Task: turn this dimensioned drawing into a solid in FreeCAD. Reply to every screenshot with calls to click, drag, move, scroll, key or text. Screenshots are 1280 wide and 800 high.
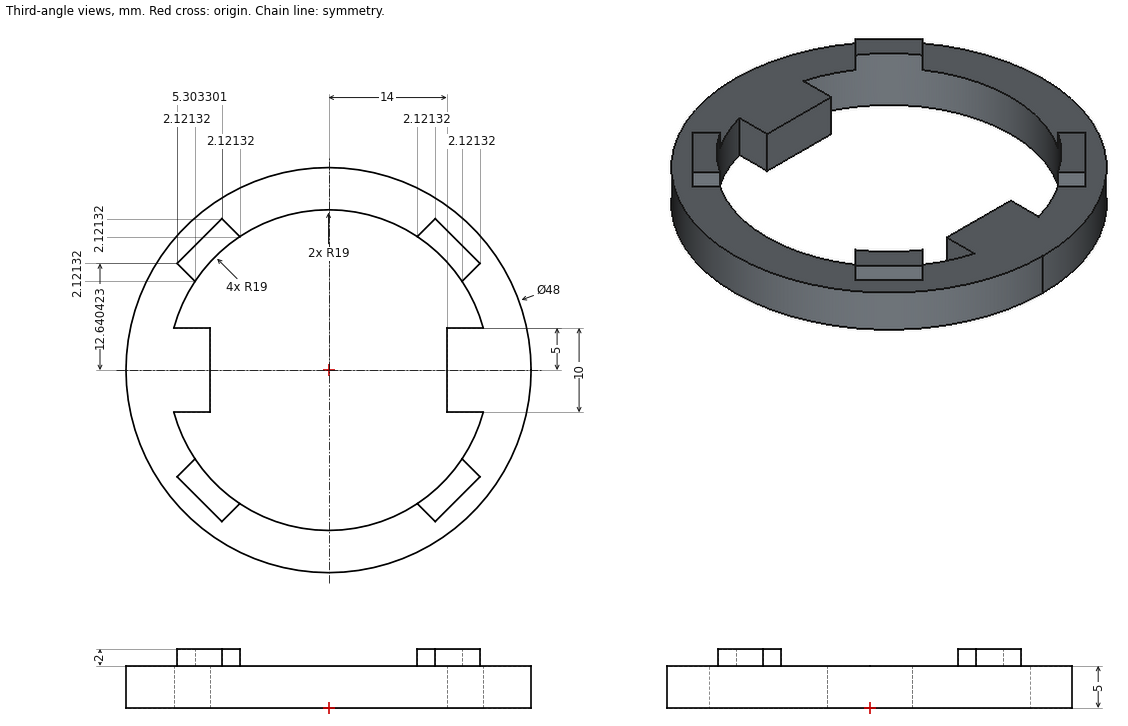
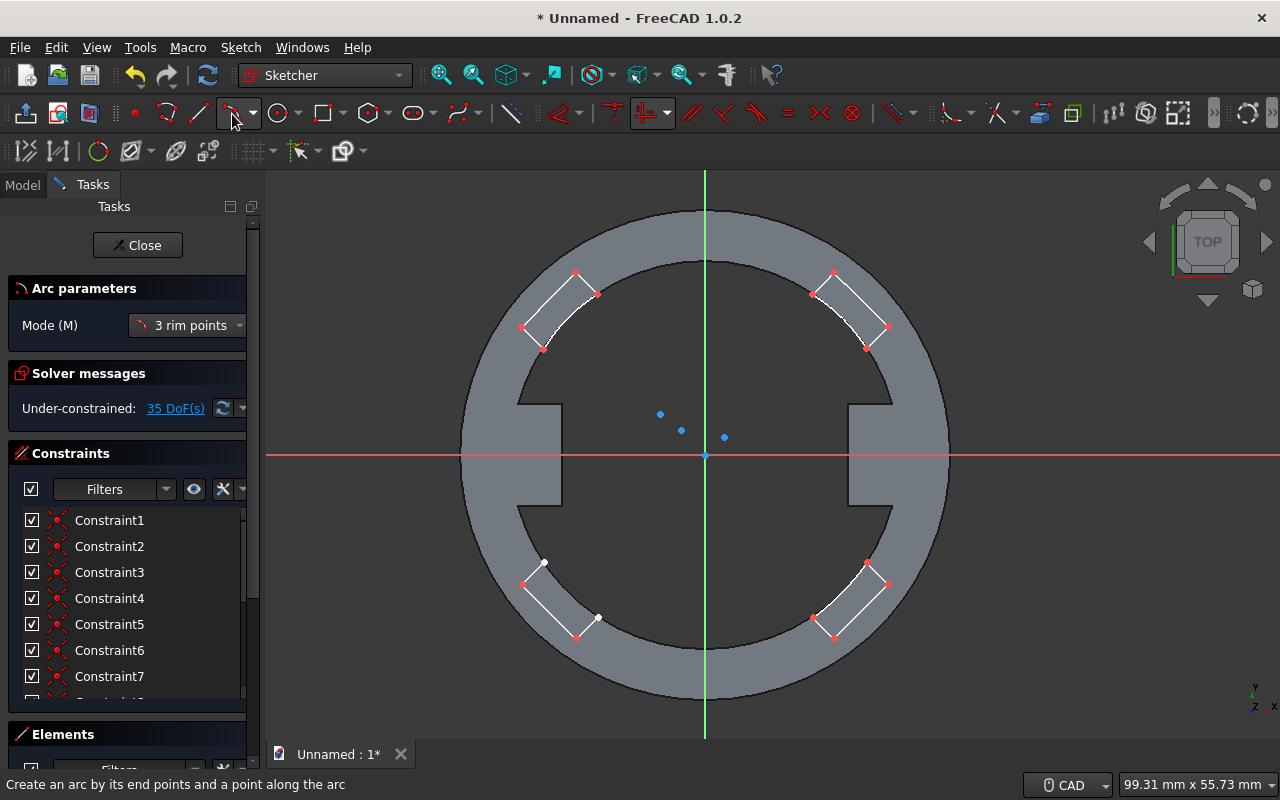
click(598, 618)
click(544, 563)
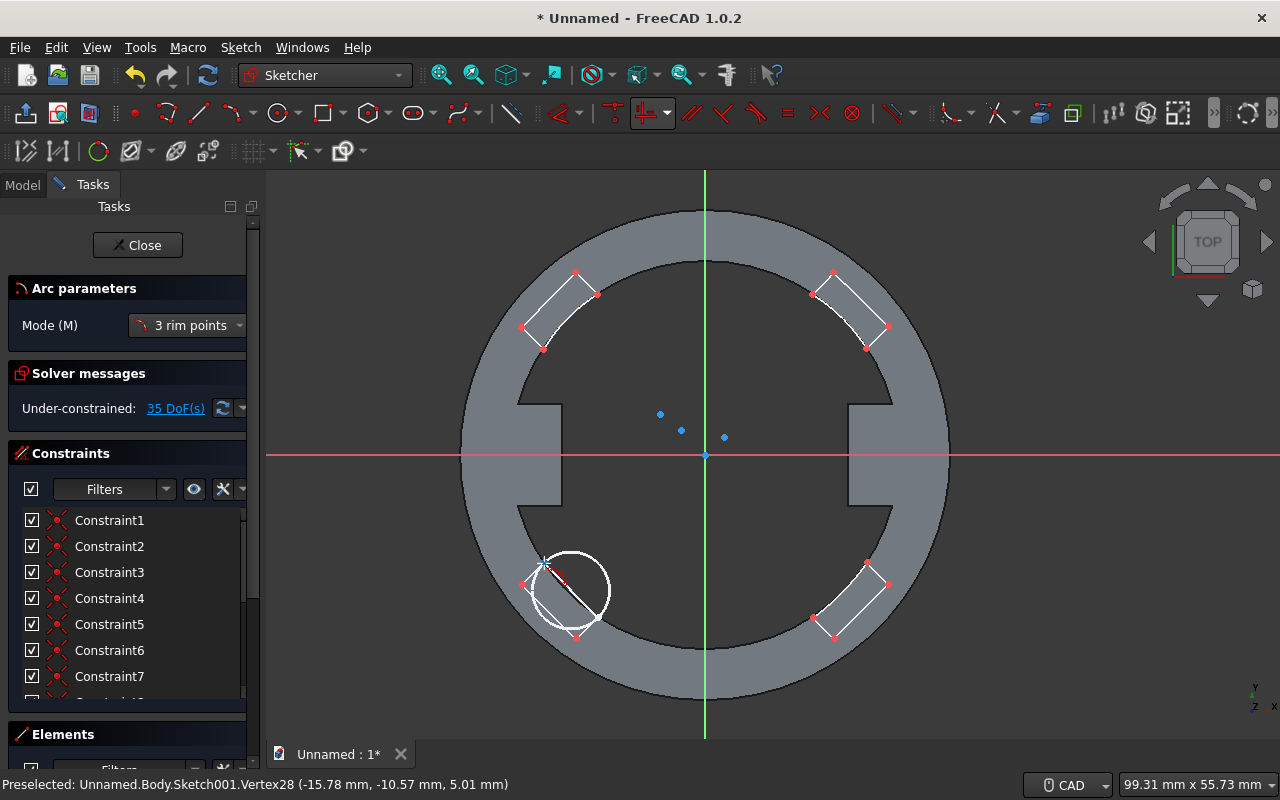
scroll(568, 592, up, 8)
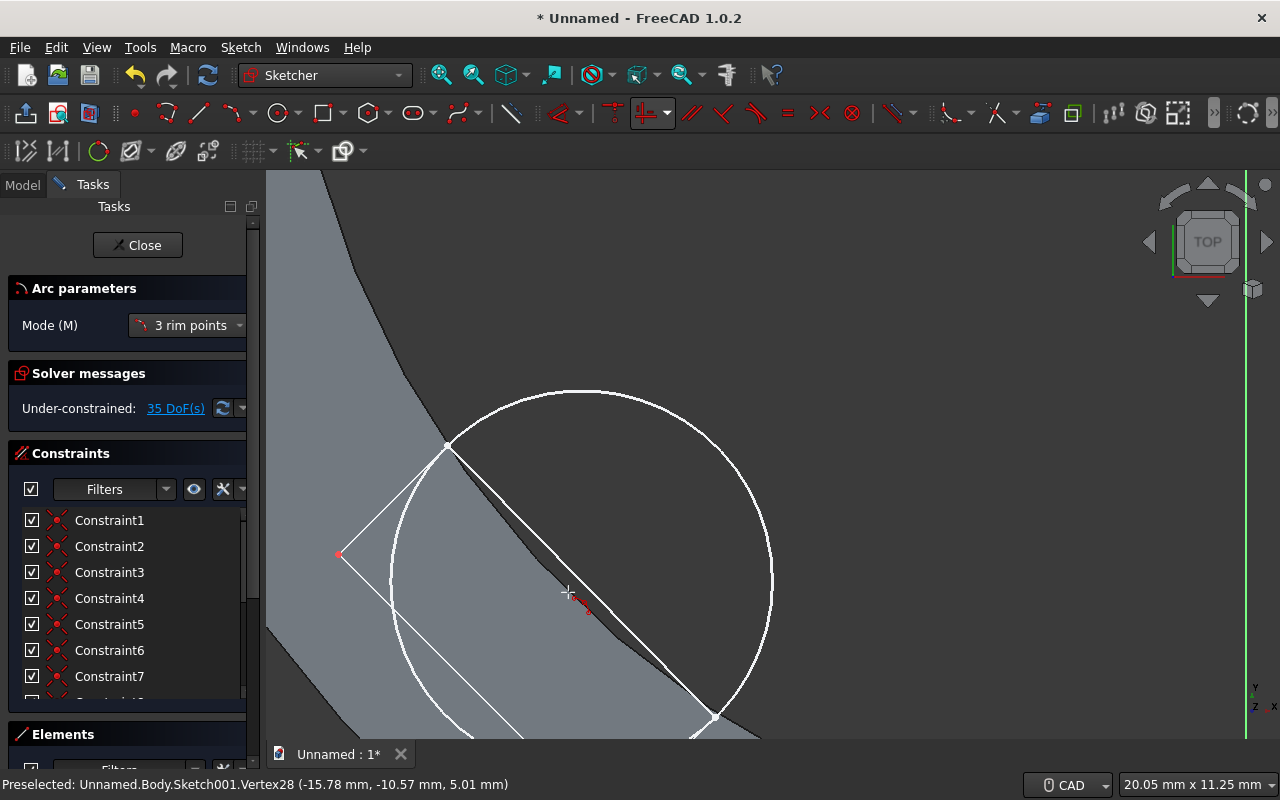
click(567, 590)
key(Escape)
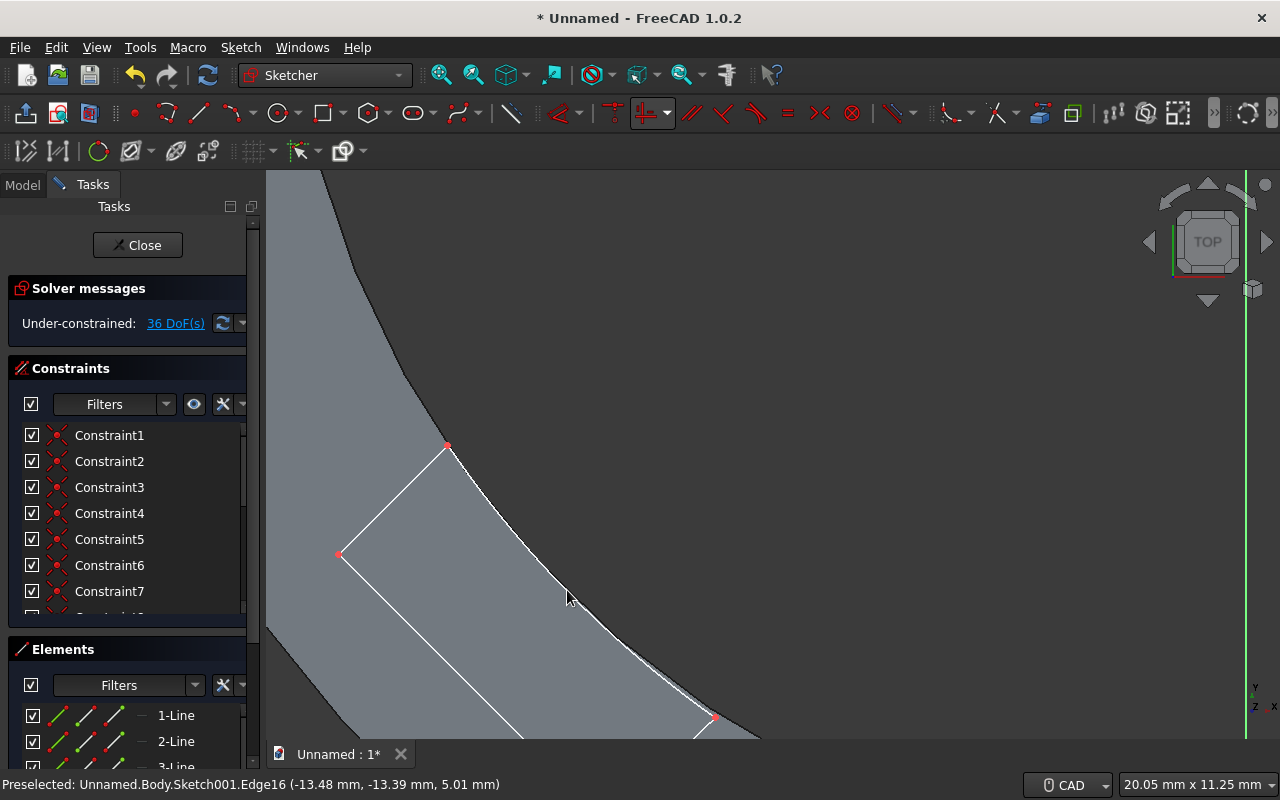
scroll(567, 592, down, 8)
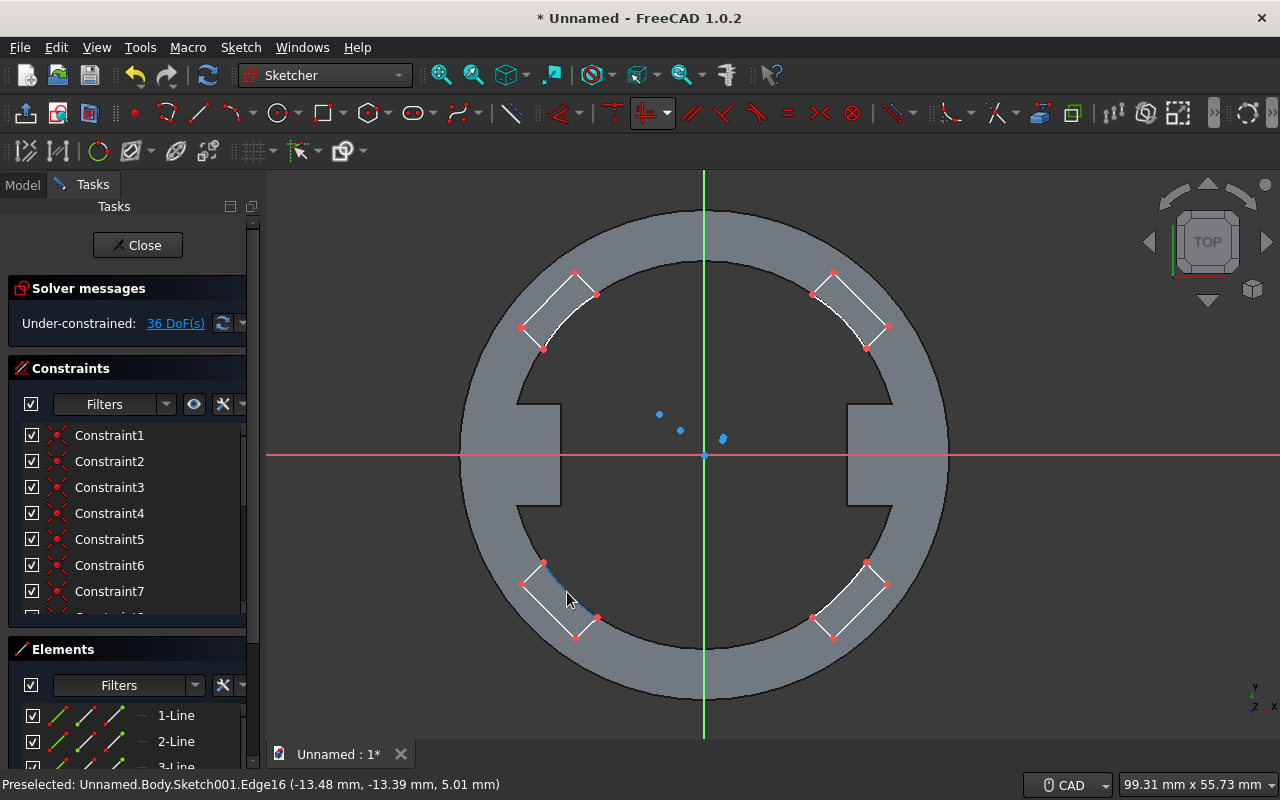
click(578, 308)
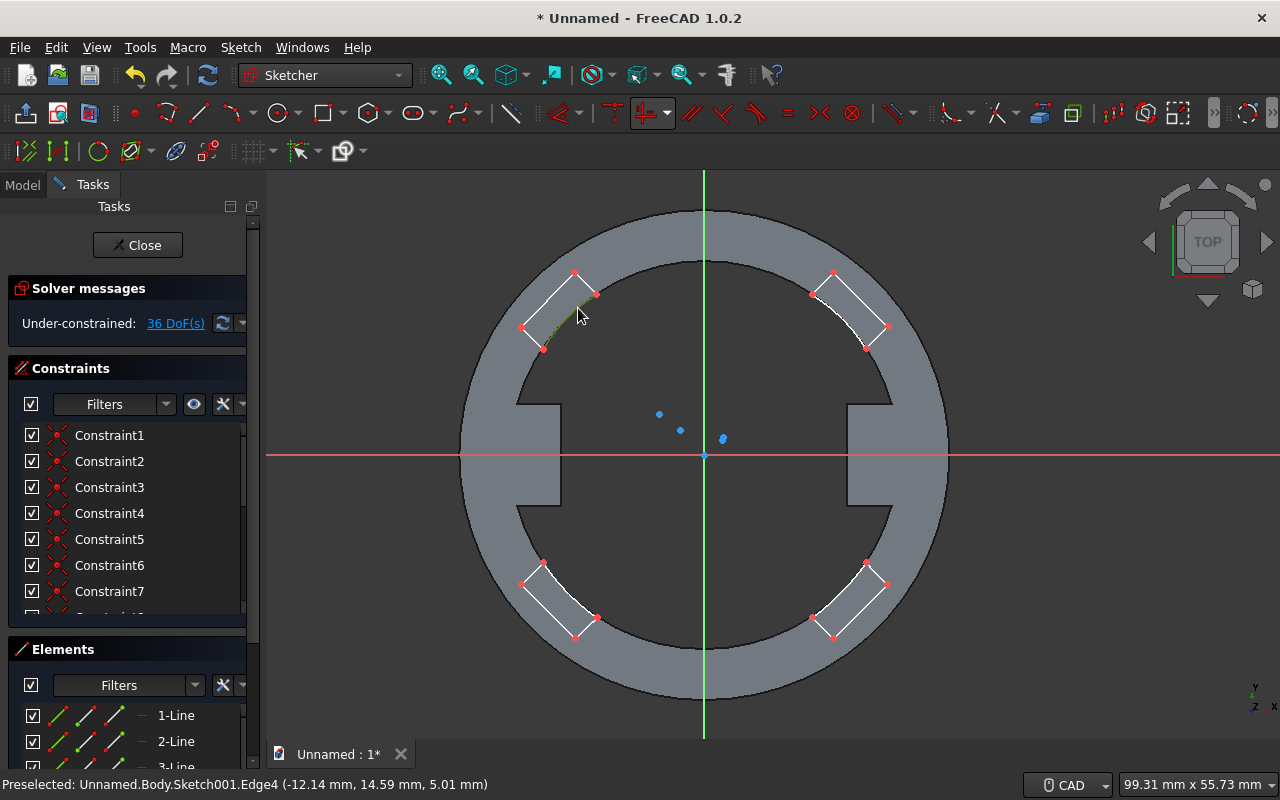
click(852, 330)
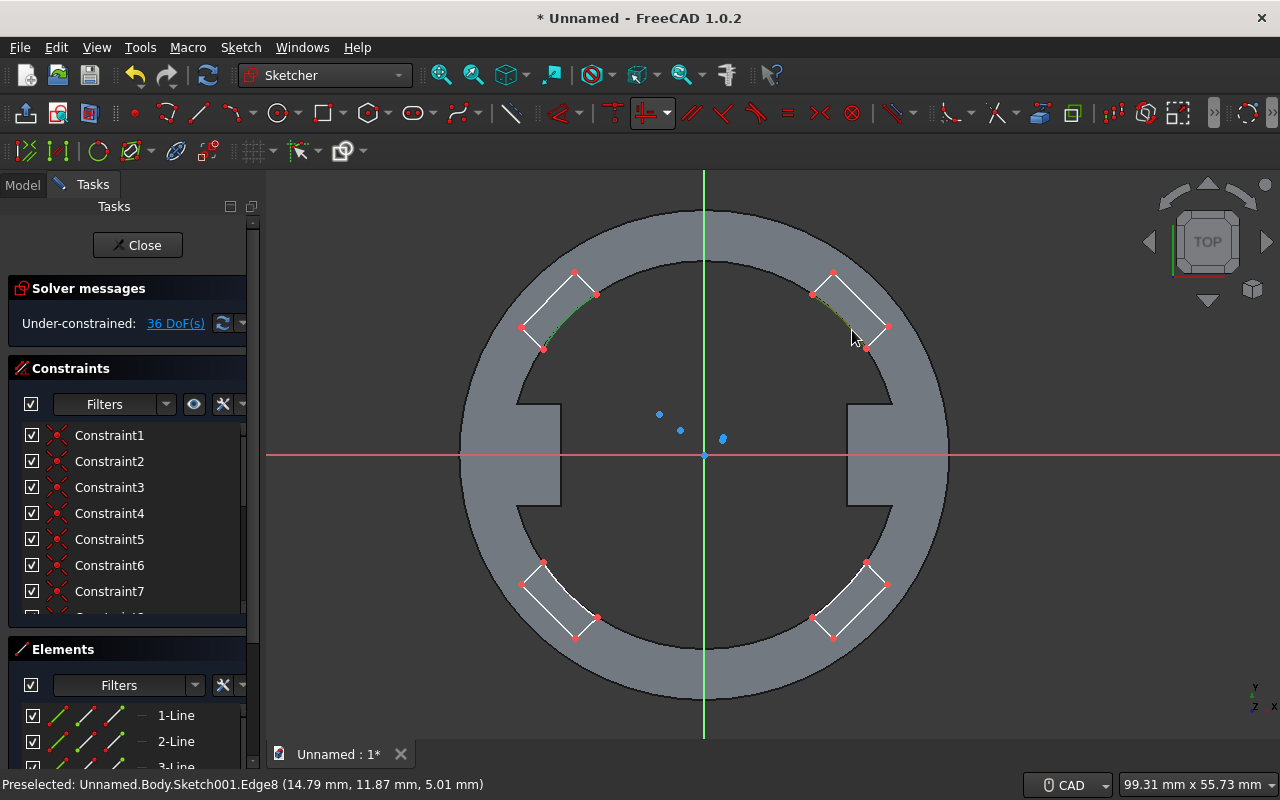
key(c)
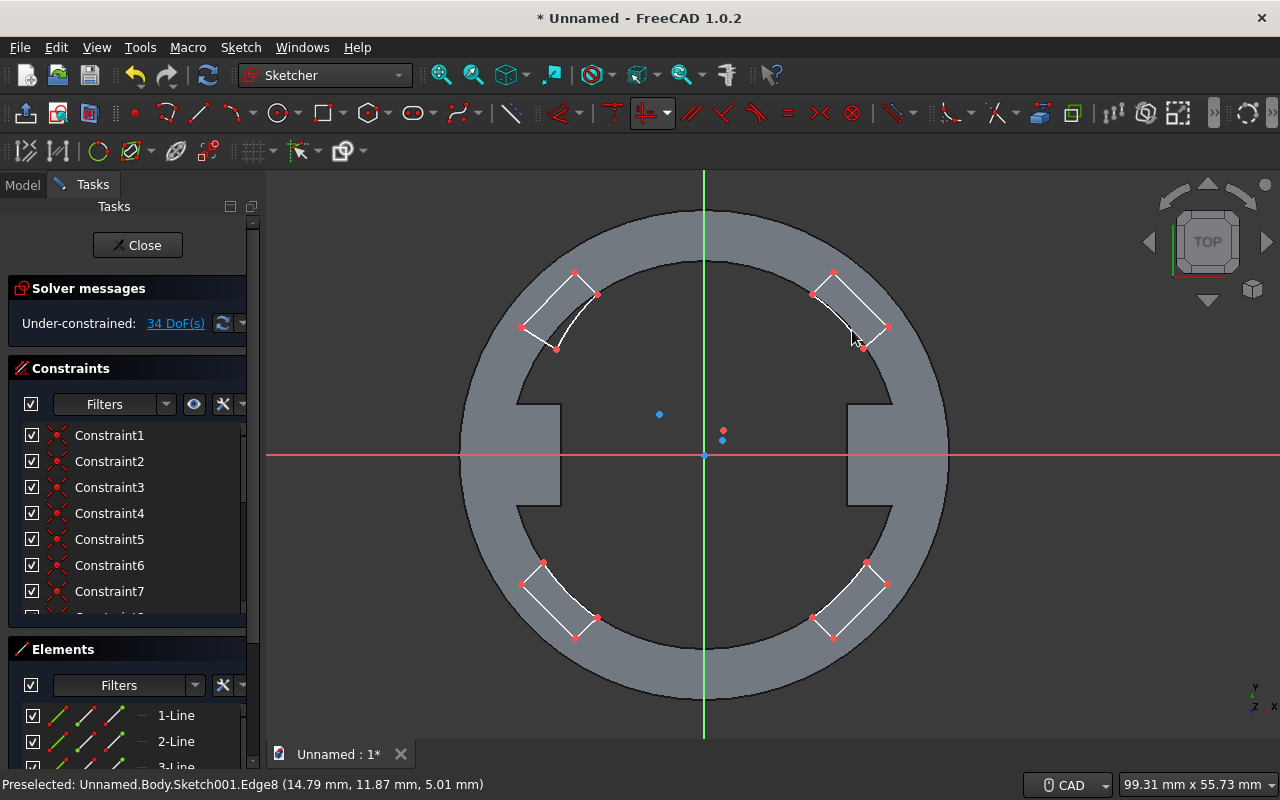
click(583, 309)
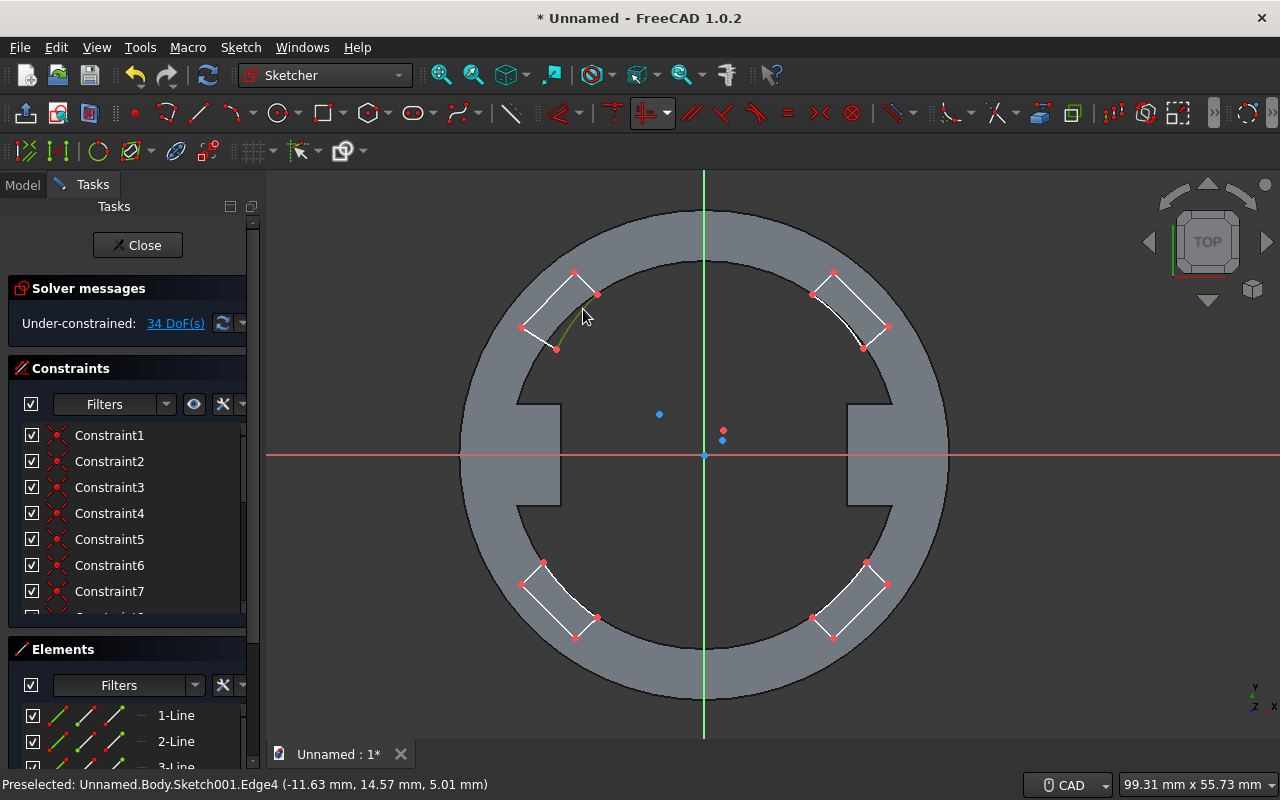
click(830, 603)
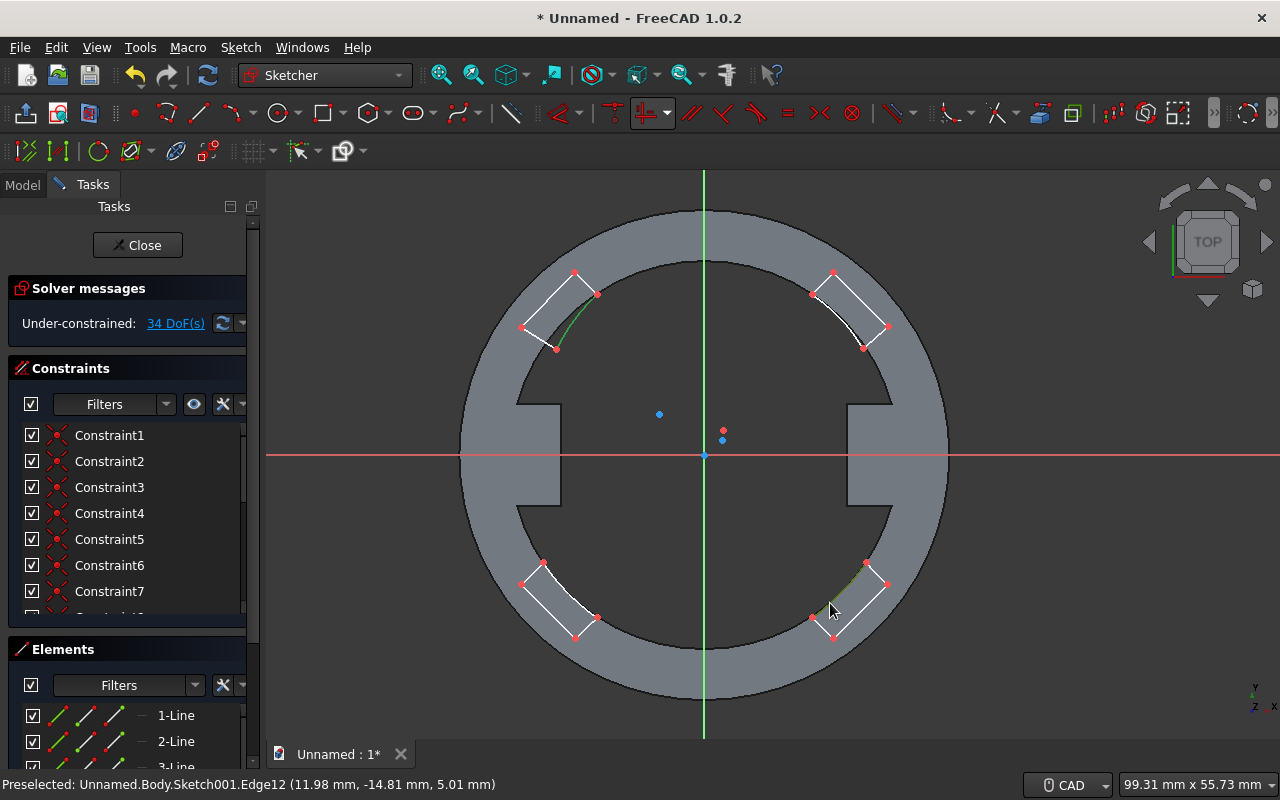
key(c)